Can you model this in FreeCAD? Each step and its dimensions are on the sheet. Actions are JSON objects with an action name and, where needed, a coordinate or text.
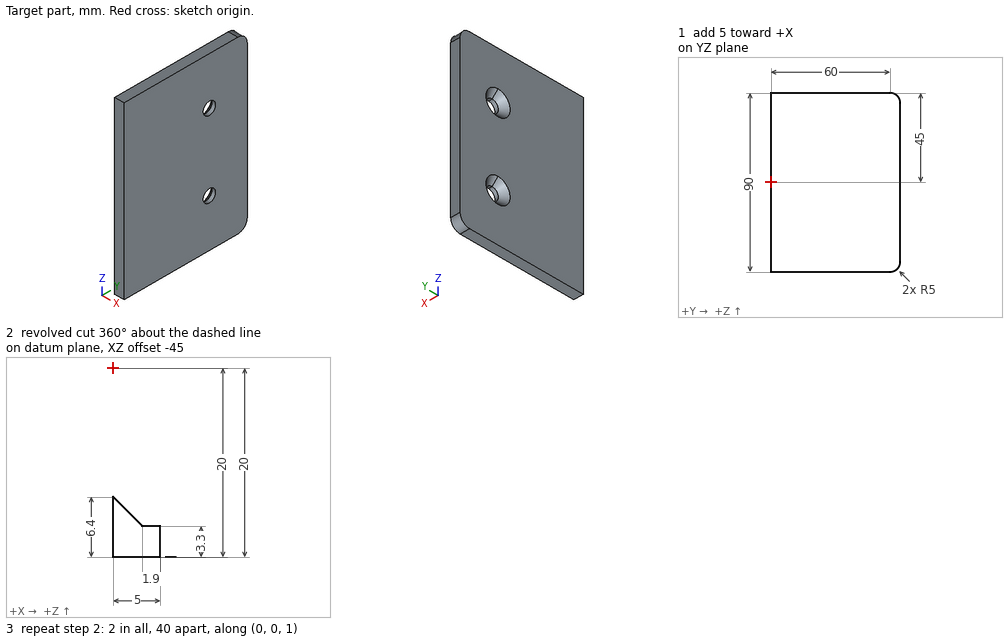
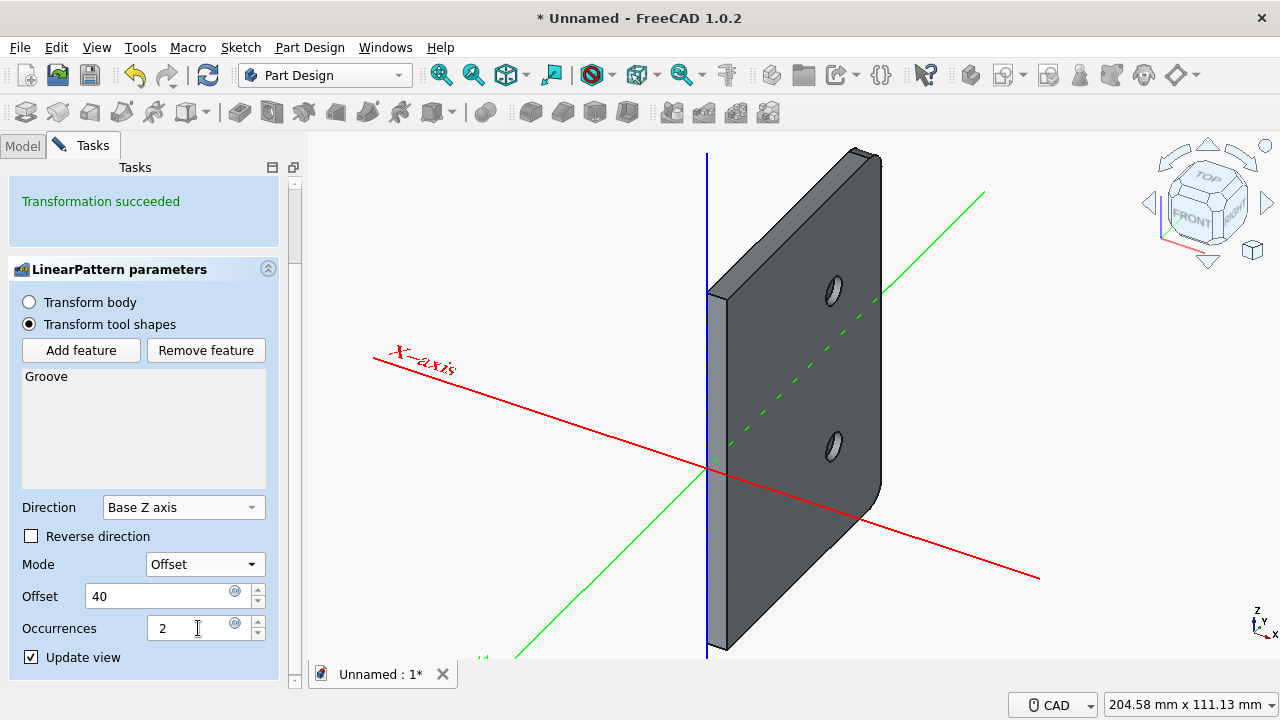
{"action": "scroll", "coordinate": [295, 432], "scroll_direction": "up", "scroll_amount": 3}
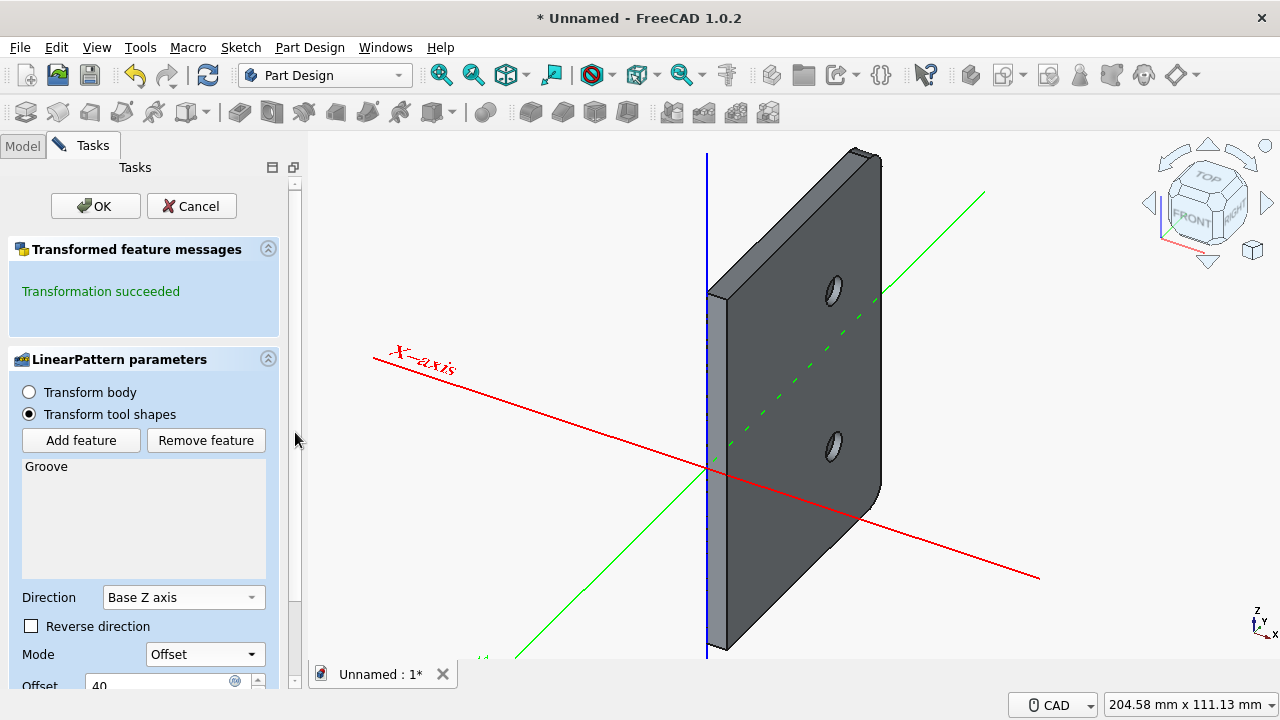
{"action": "left_click", "coordinate": [96, 206]}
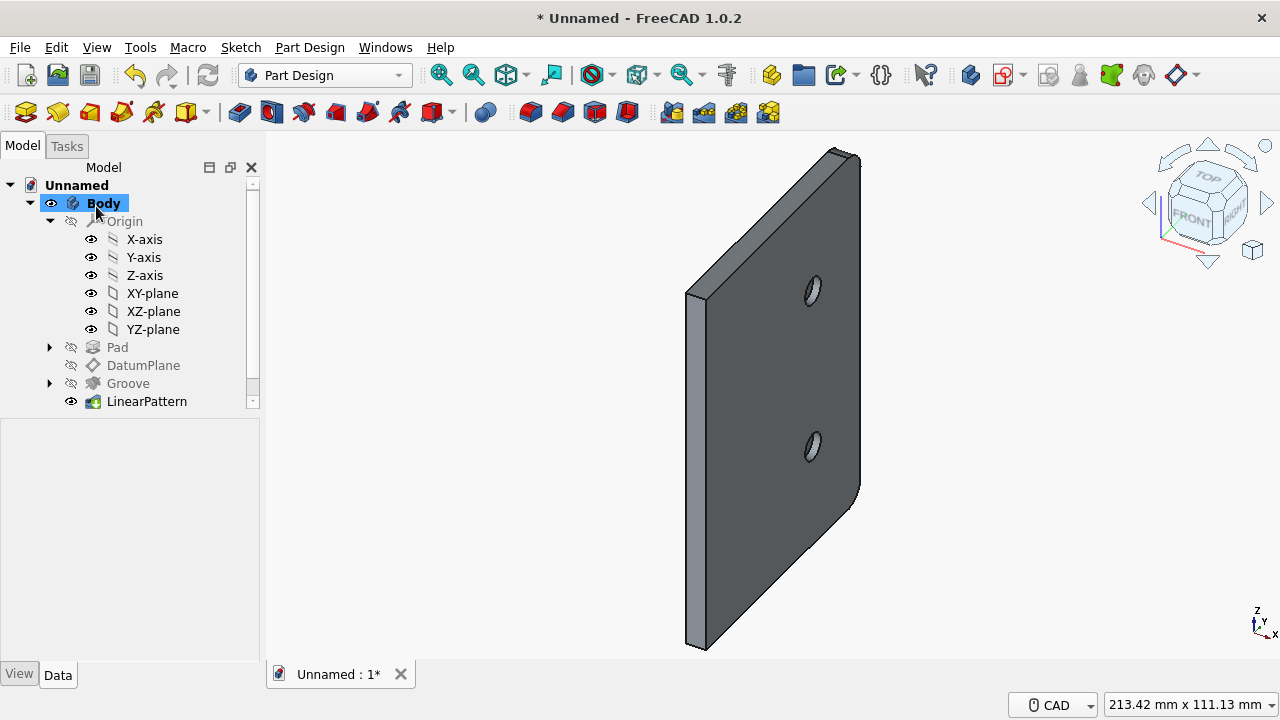
{"action": "key", "text": "0"}